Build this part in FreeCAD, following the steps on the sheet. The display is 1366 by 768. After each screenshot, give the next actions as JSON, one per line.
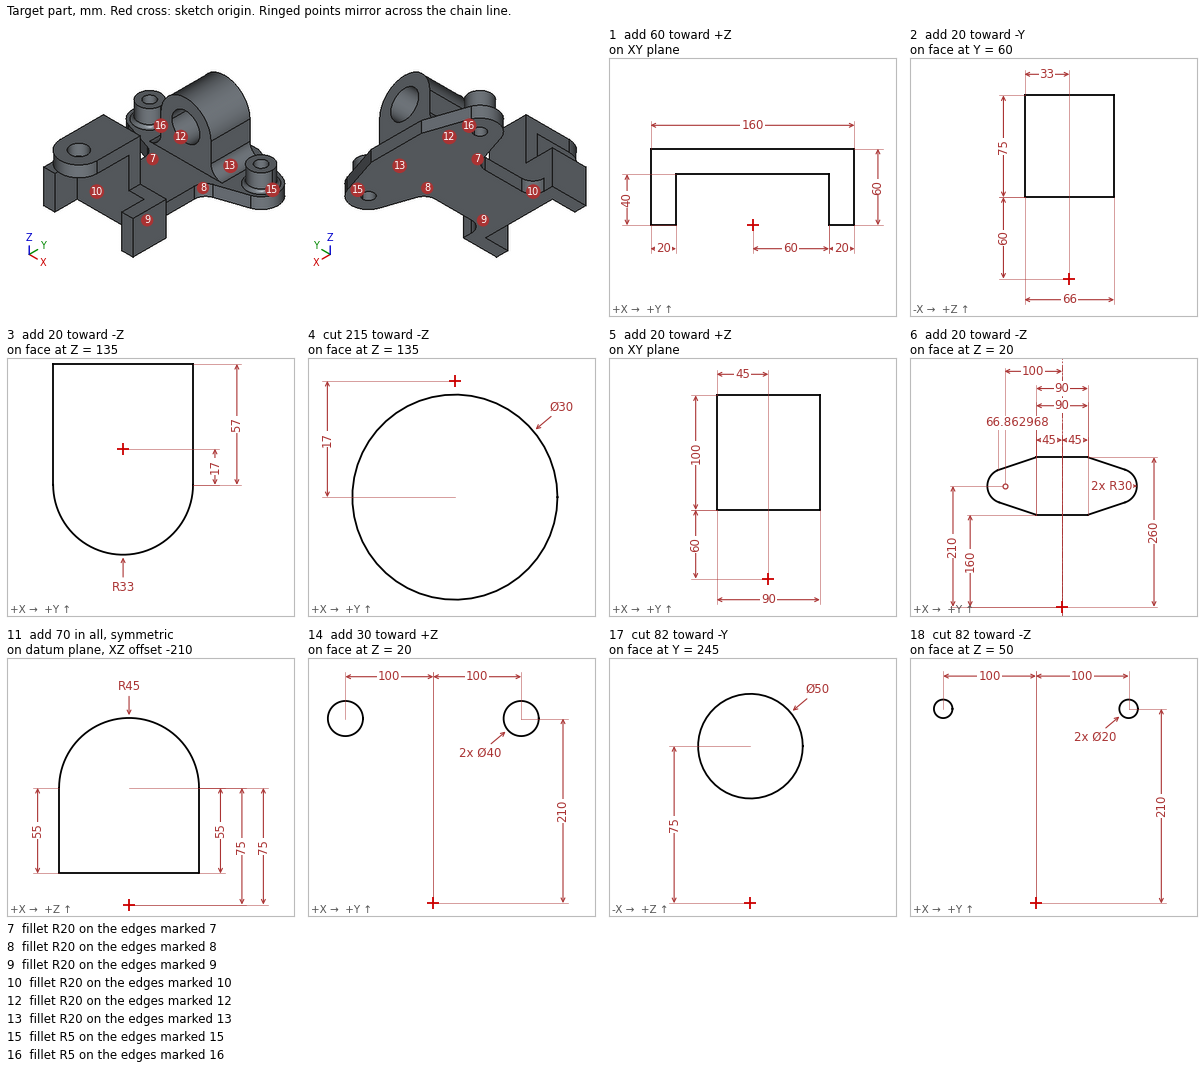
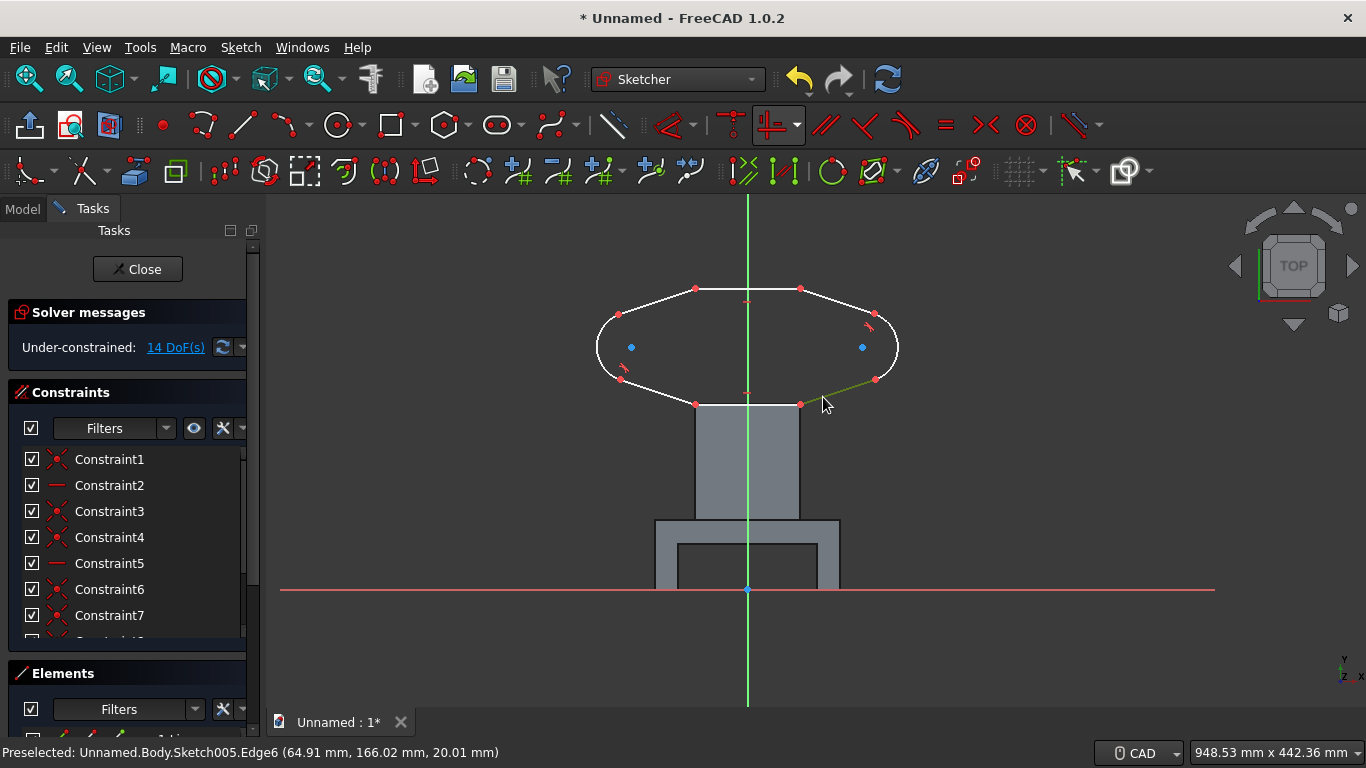
{"action": "left_click", "coordinate": [894, 363]}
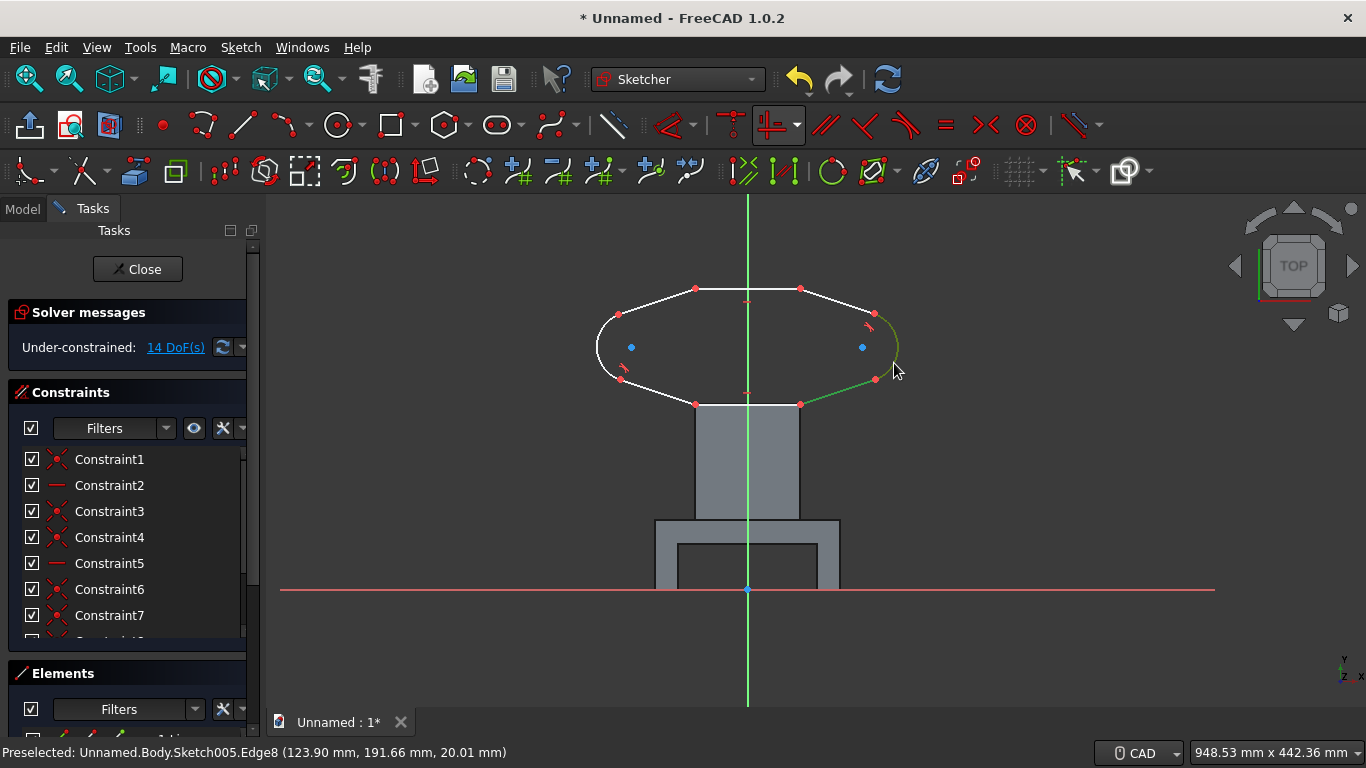
{"action": "key", "text": "t"}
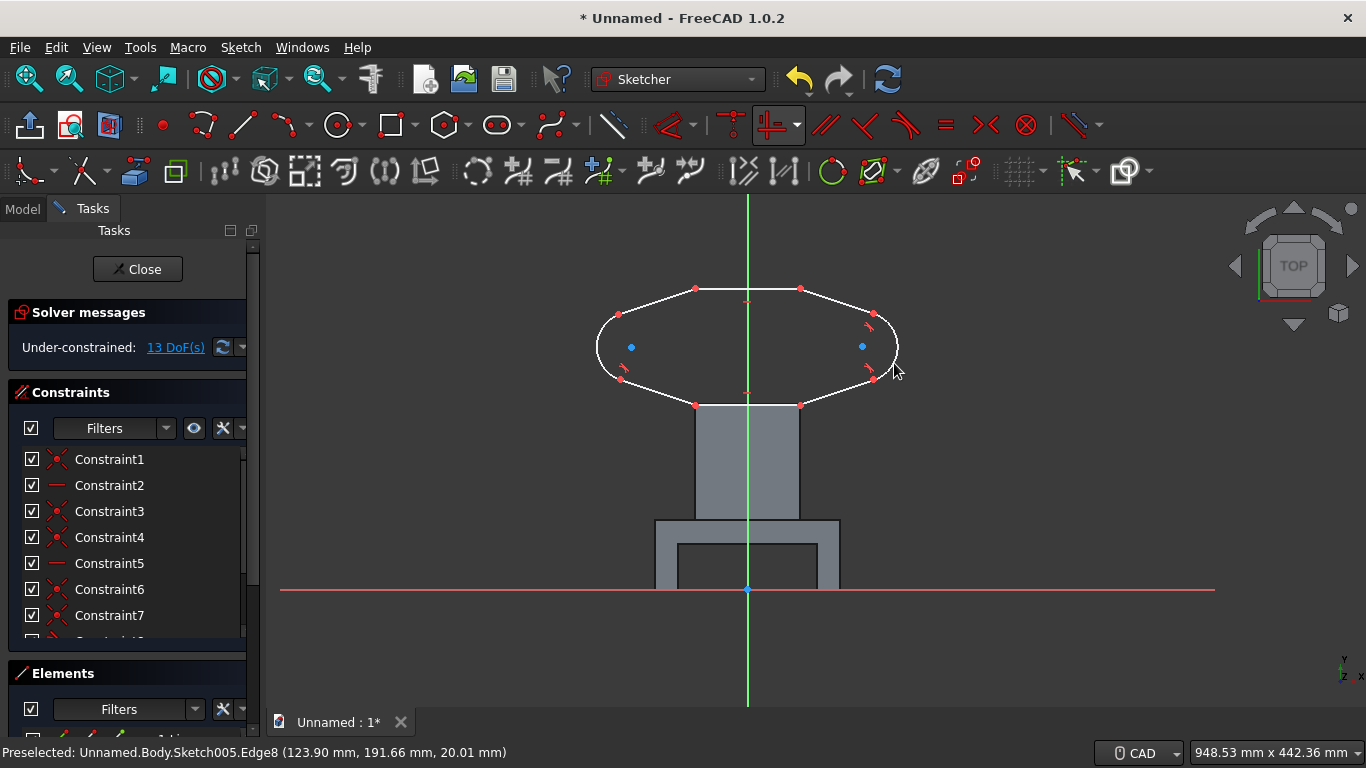
{"action": "left_click", "coordinate": [600, 332]}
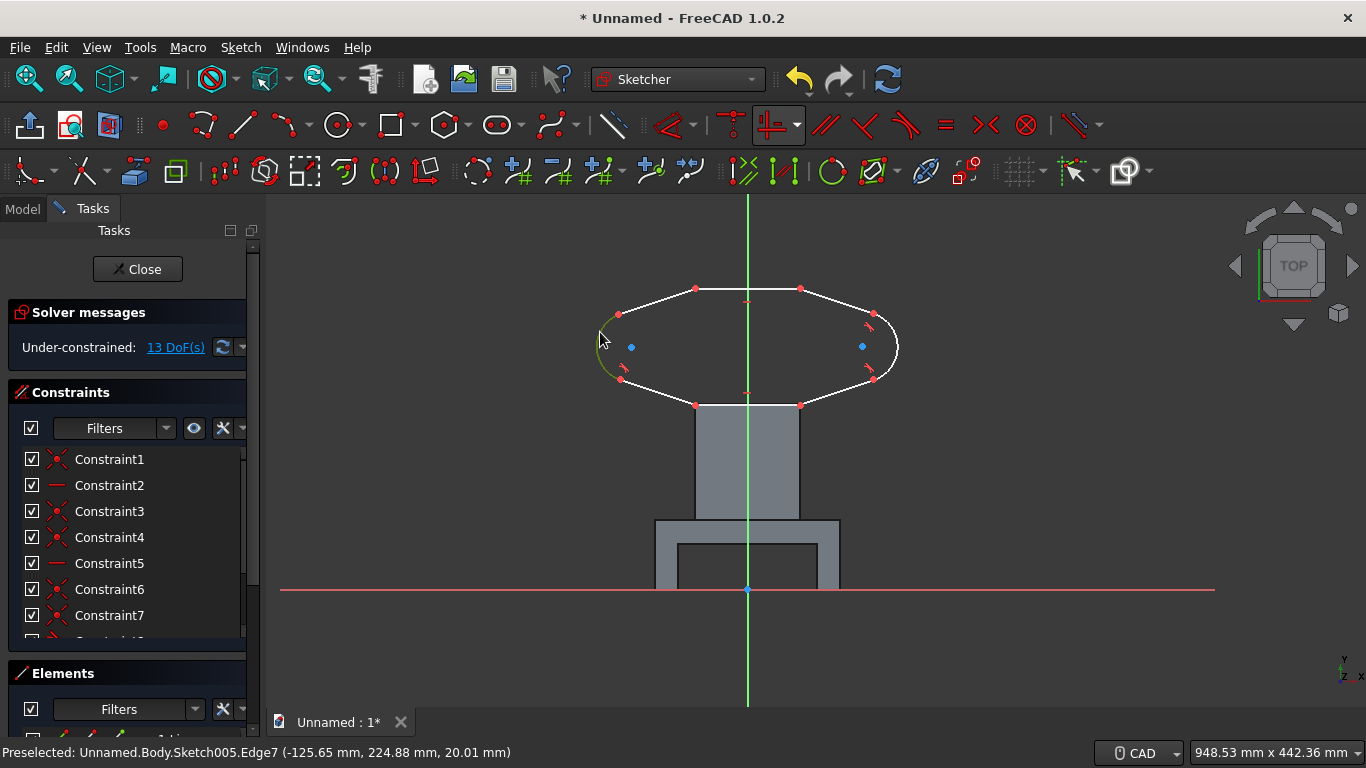
{"action": "left_click", "coordinate": [893, 364]}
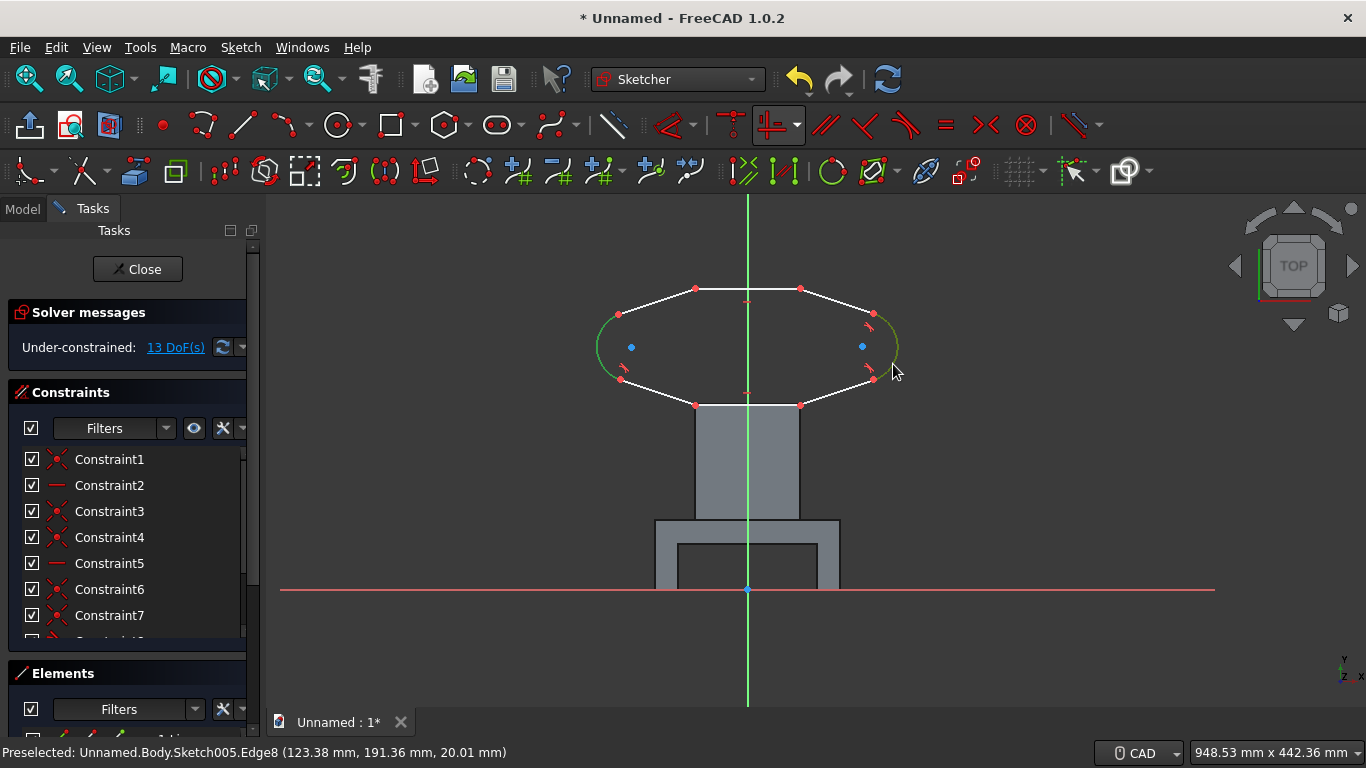
{"action": "key", "text": "e"}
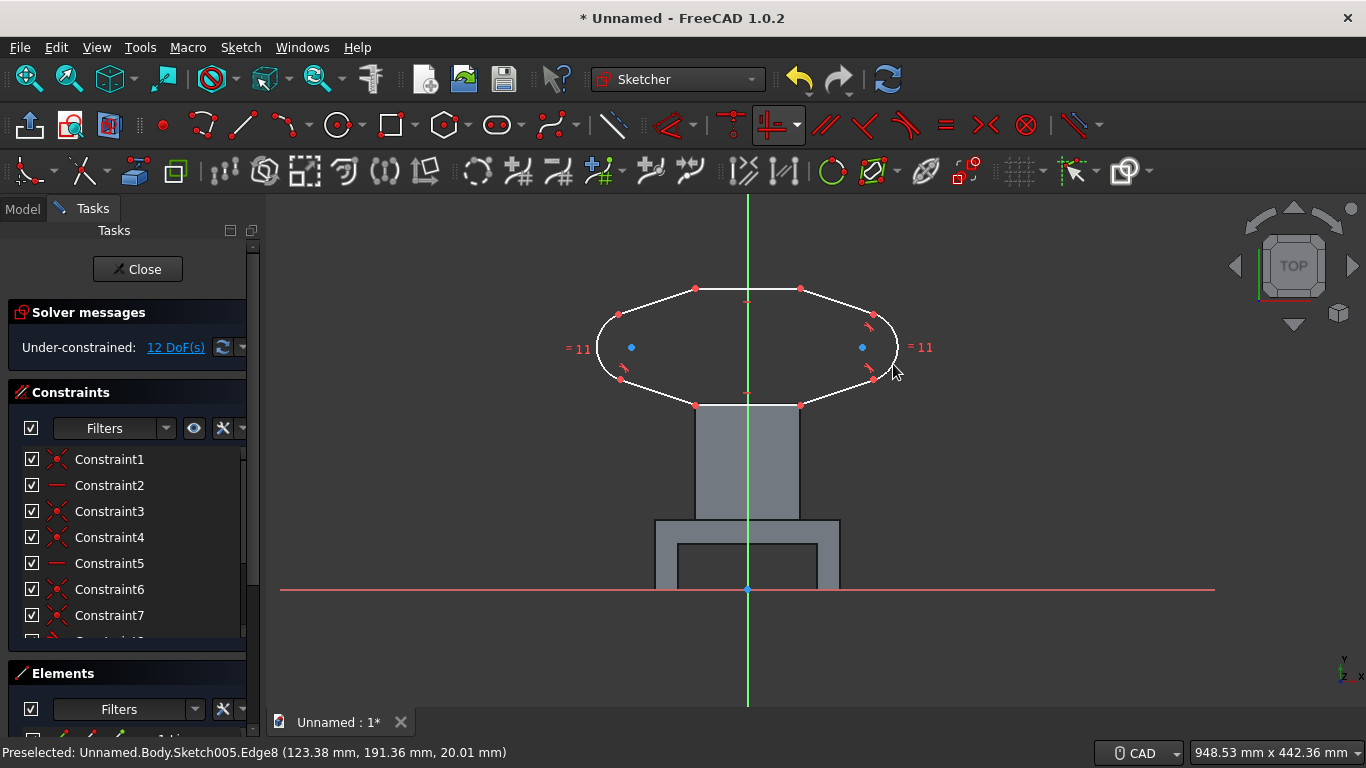
{"action": "left_click", "coordinate": [632, 347]}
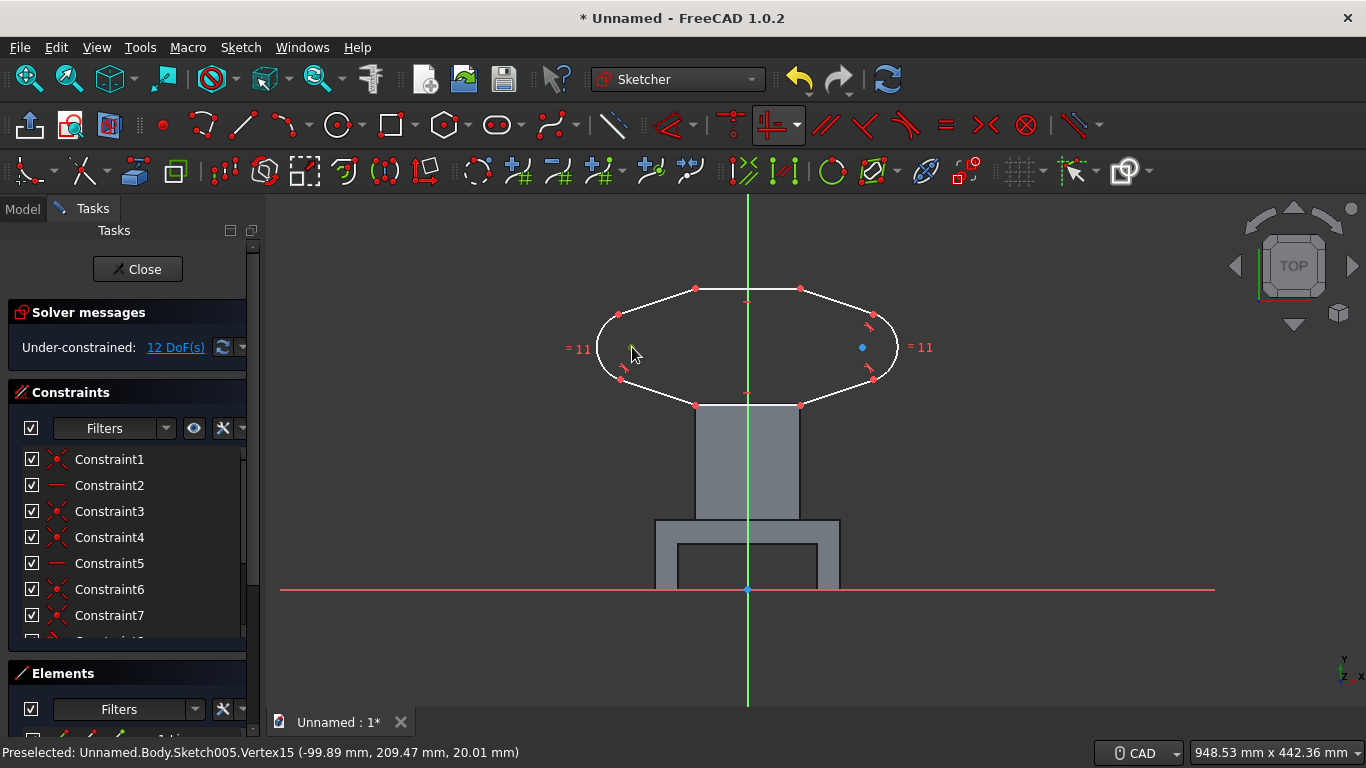
{"action": "left_click", "coordinate": [863, 347]}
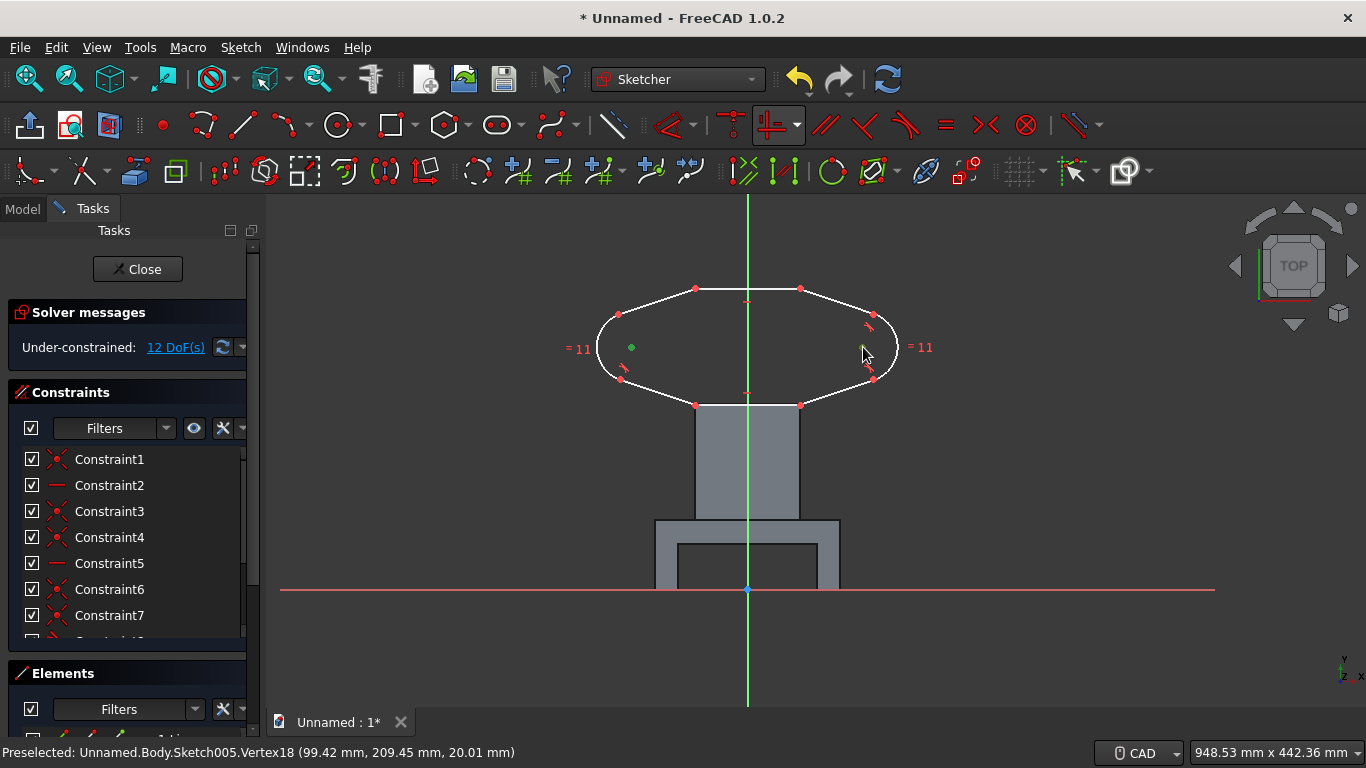
{"action": "left_click", "coordinate": [748, 646]}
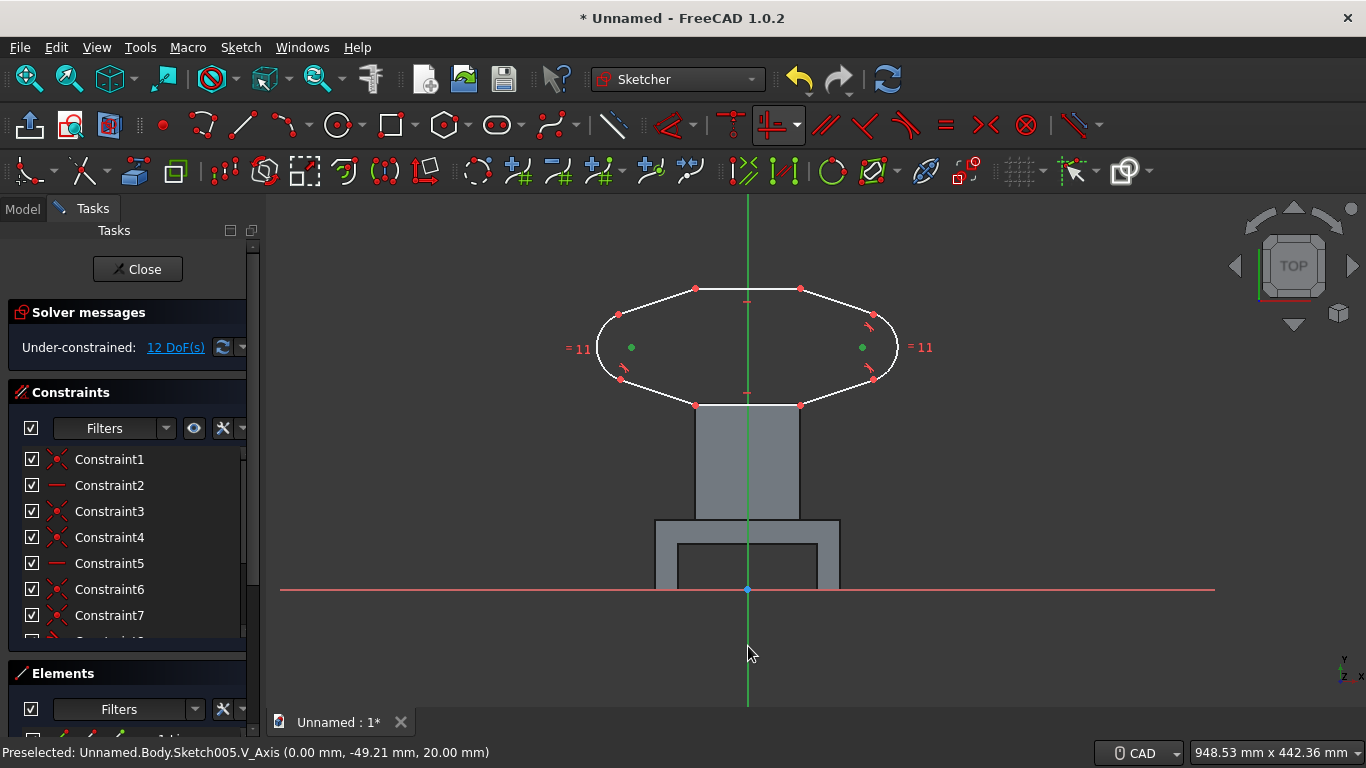
{"action": "left_click", "coordinate": [986, 126]}